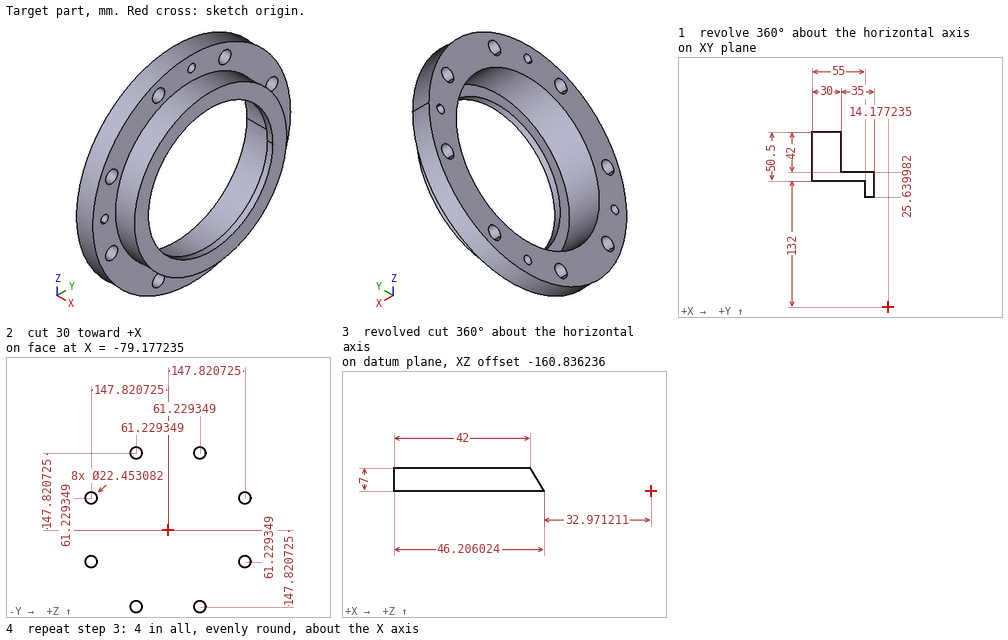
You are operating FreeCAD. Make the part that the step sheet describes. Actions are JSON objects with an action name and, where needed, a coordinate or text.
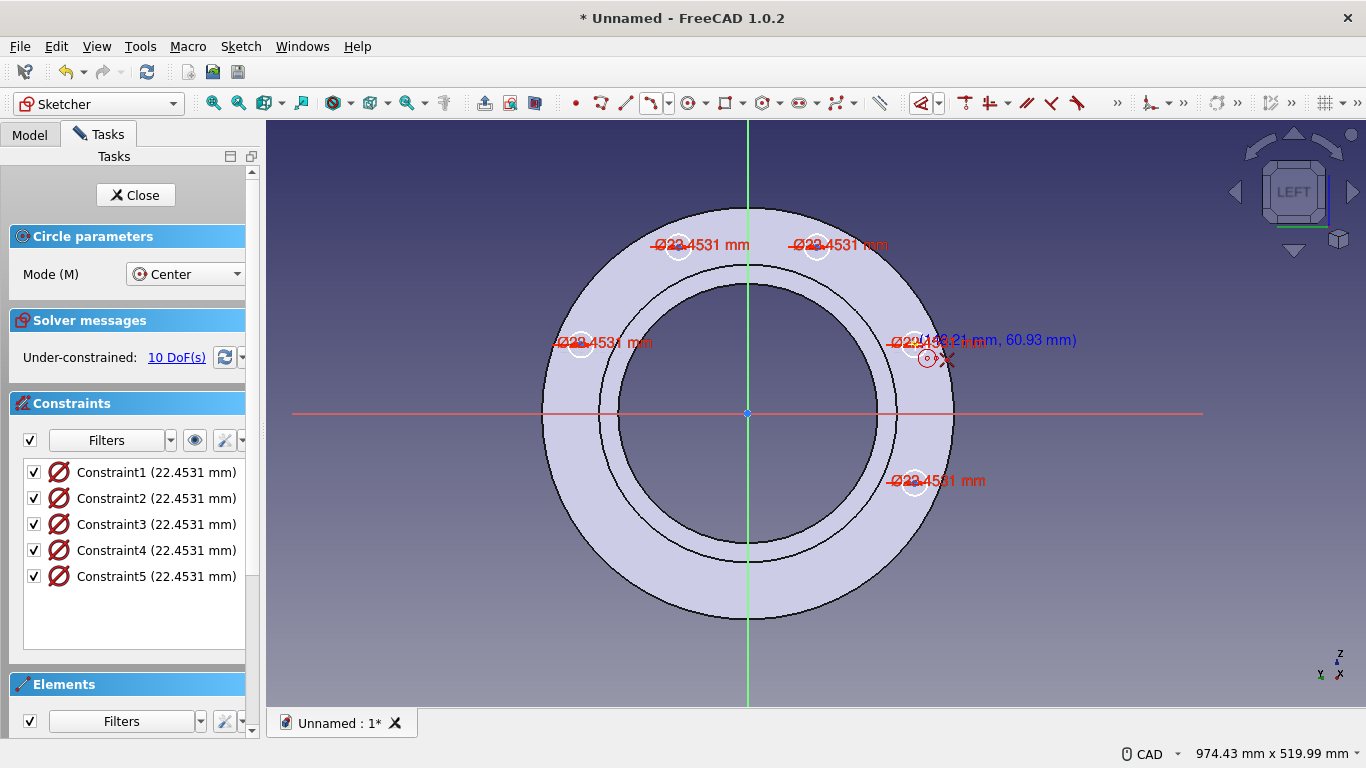
{"action": "scroll", "coordinate": [817, 580], "scroll_direction": "up", "scroll_amount": 3}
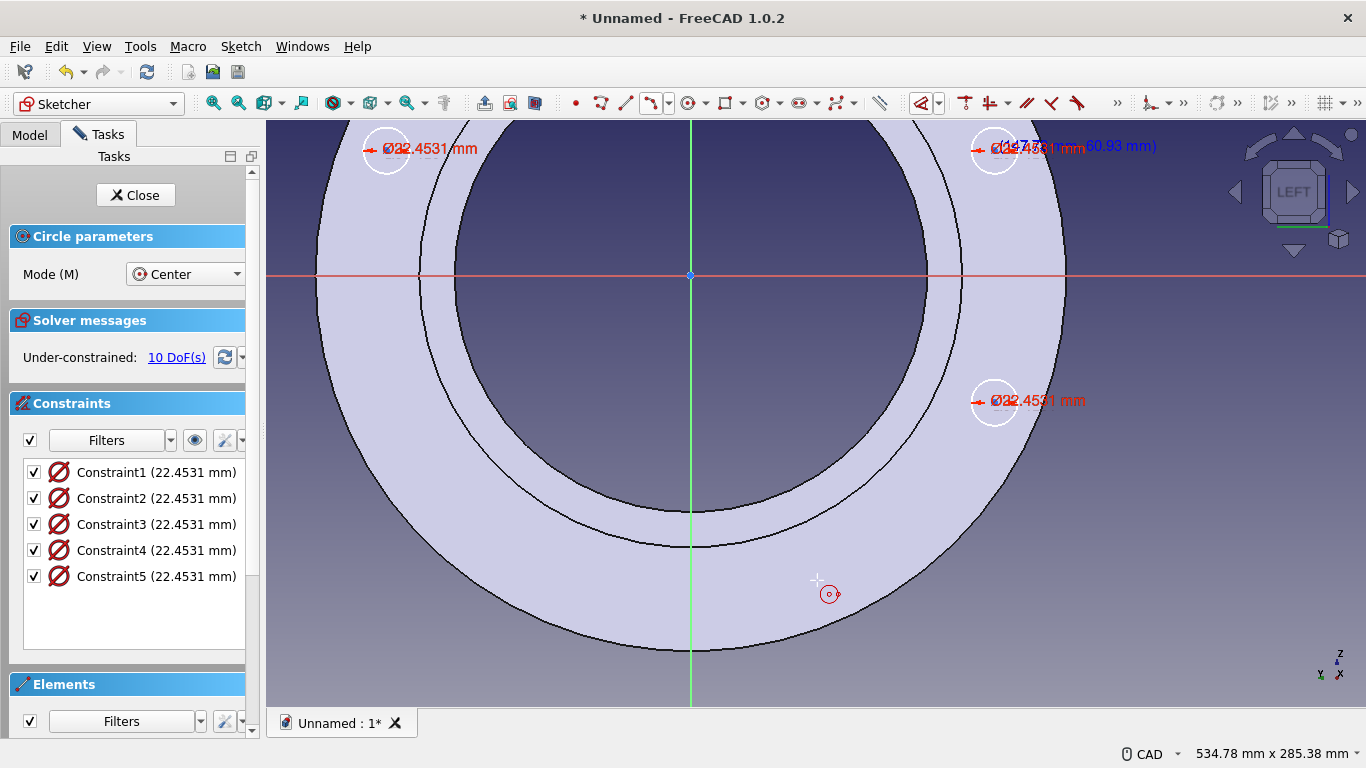
{"action": "left_click", "coordinate": [817, 580]}
{"action": "mouse_move", "coordinate": [833, 564]}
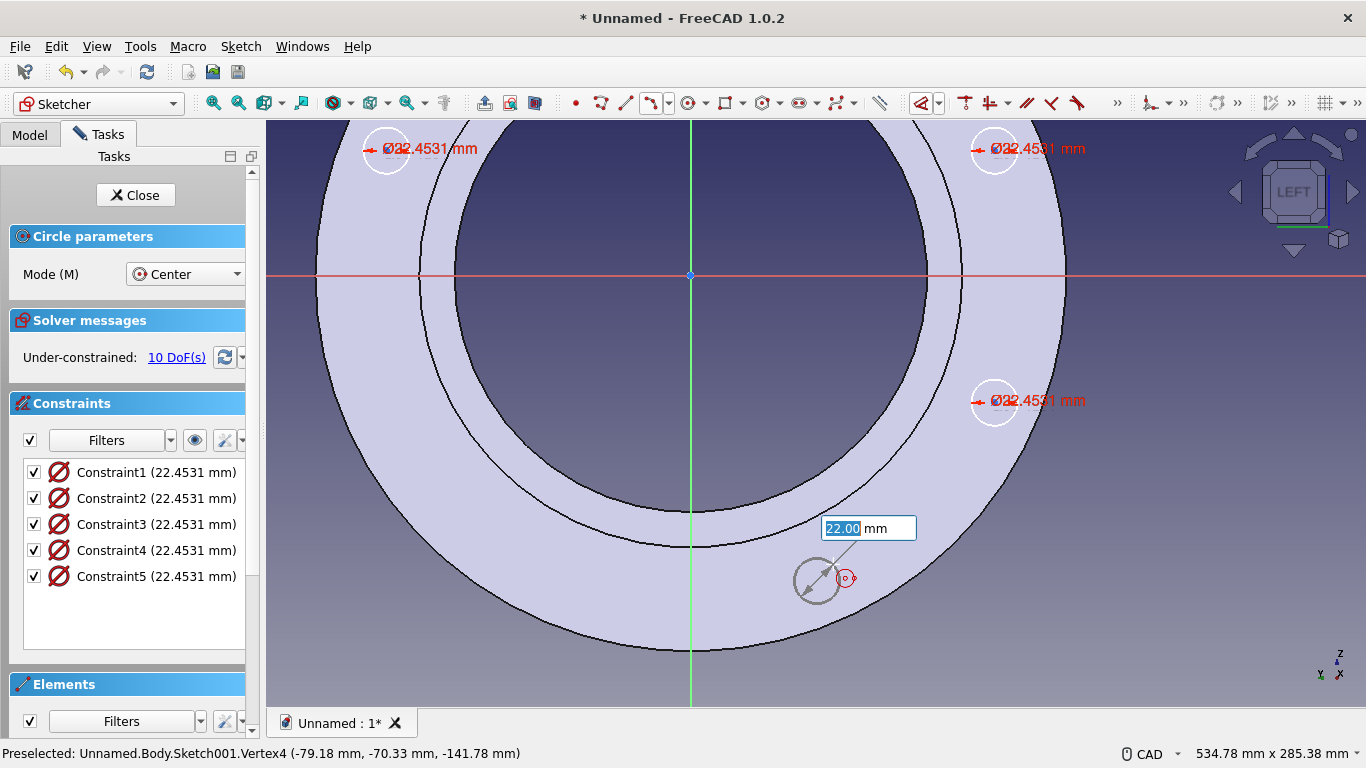
{"action": "type", "text": "22.453082"}
{"action": "key", "text": "Return"}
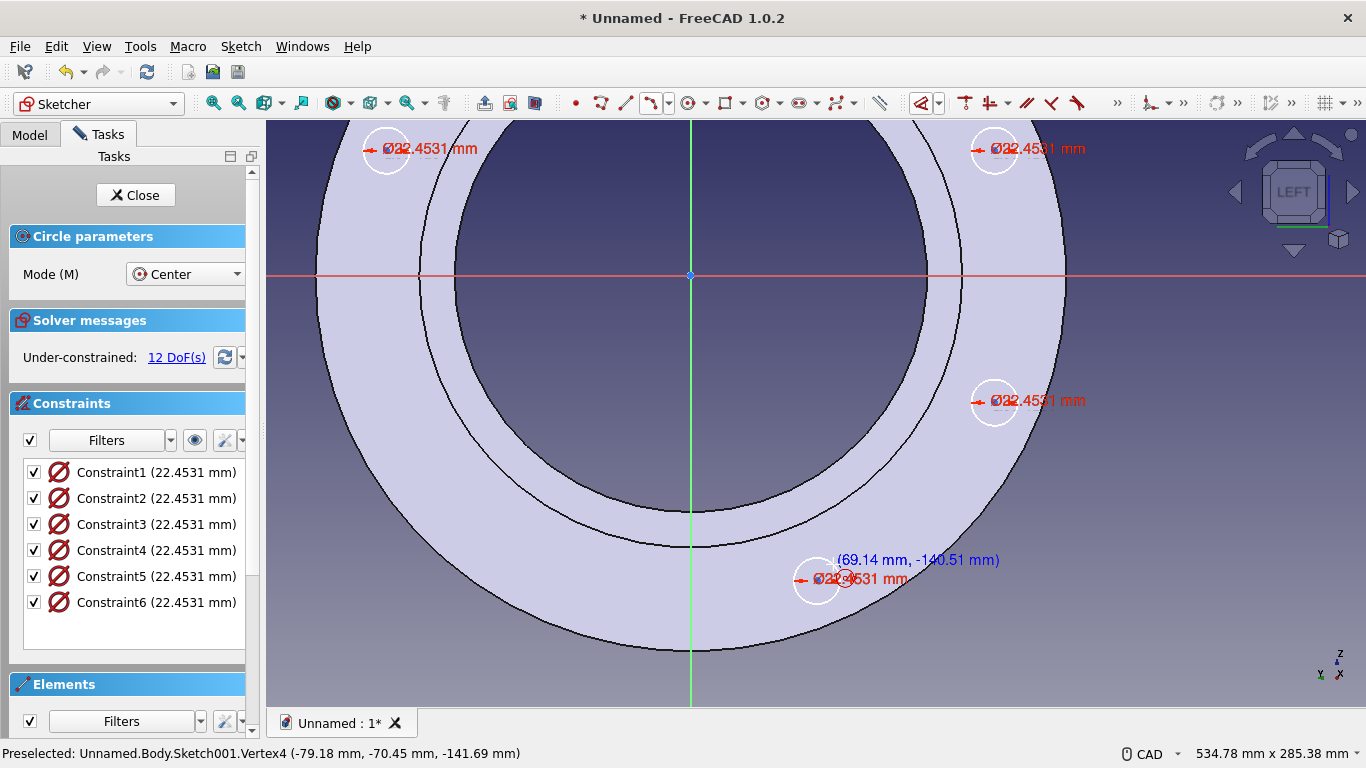
{"action": "left_click", "coordinate": [565, 580]}
{"action": "mouse_move", "coordinate": [581, 564]}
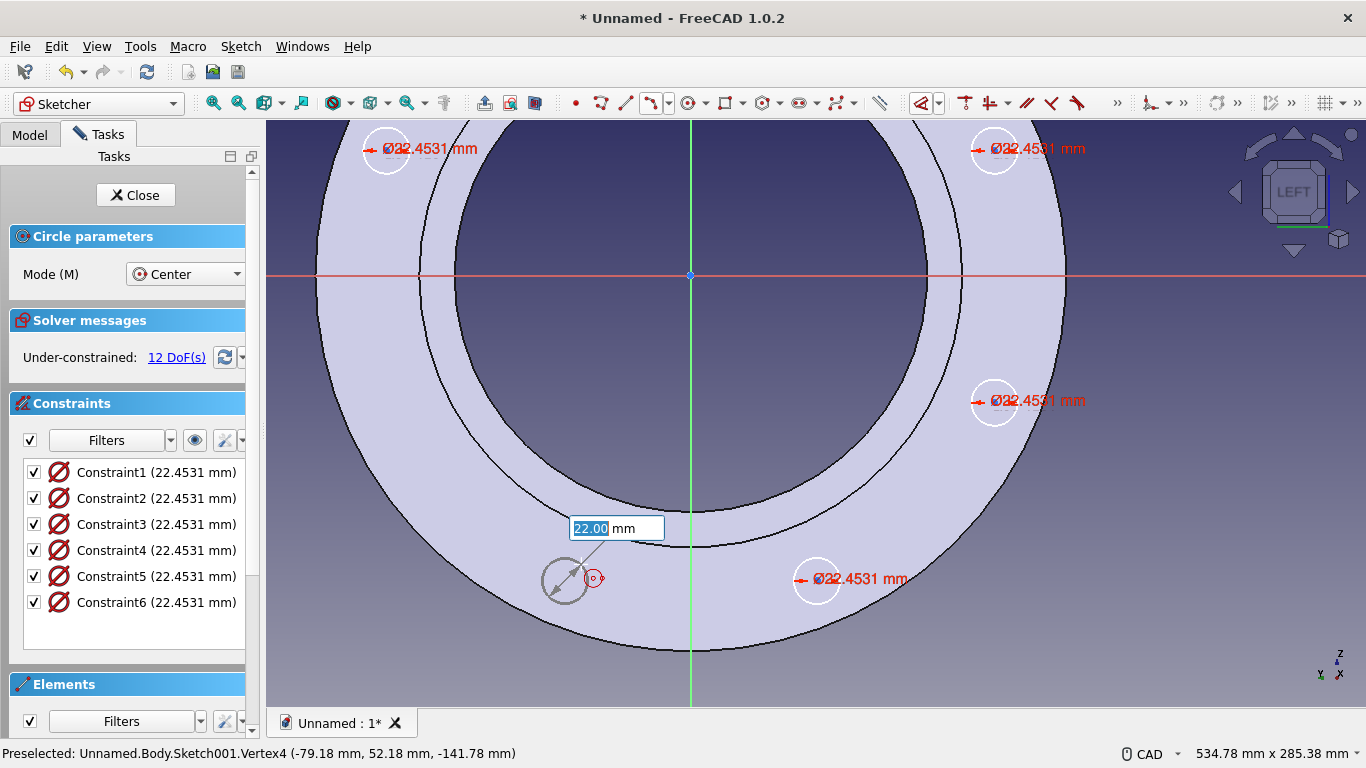
{"action": "type", "text": "22.453082"}
{"action": "key", "text": "Return"}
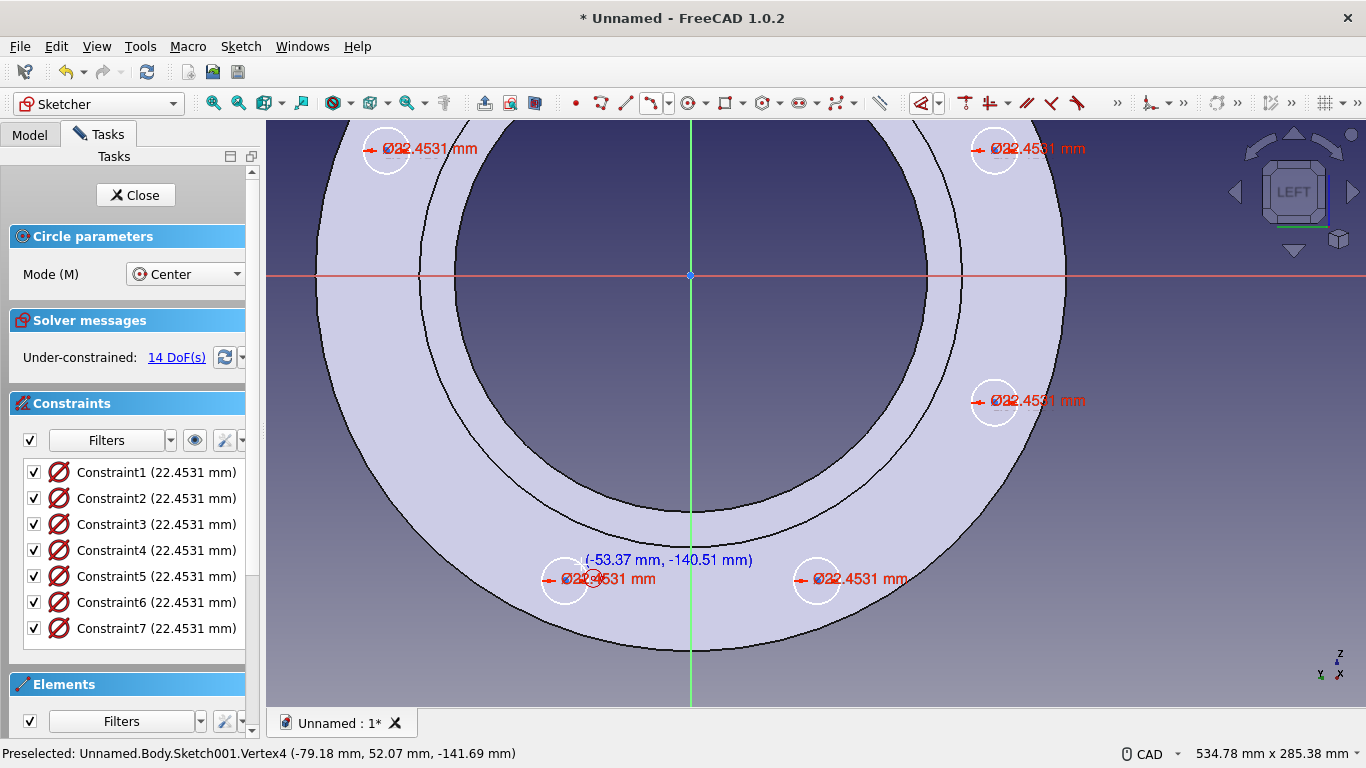
{"action": "left_click", "coordinate": [387, 402]}
{"action": "mouse_move", "coordinate": [403, 386]}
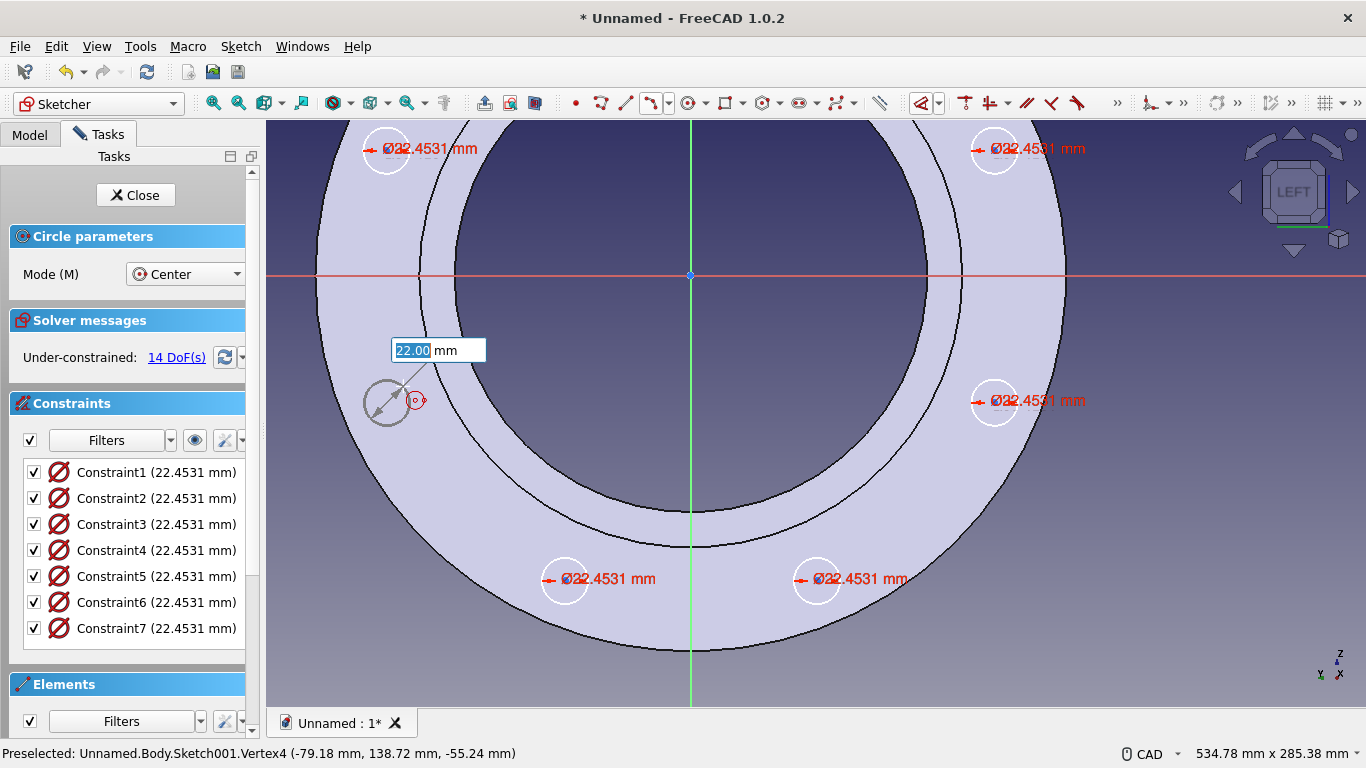
{"action": "type", "text": "22.453082"}
{"action": "key", "text": "Return"}
{"action": "key", "text": "Escape"}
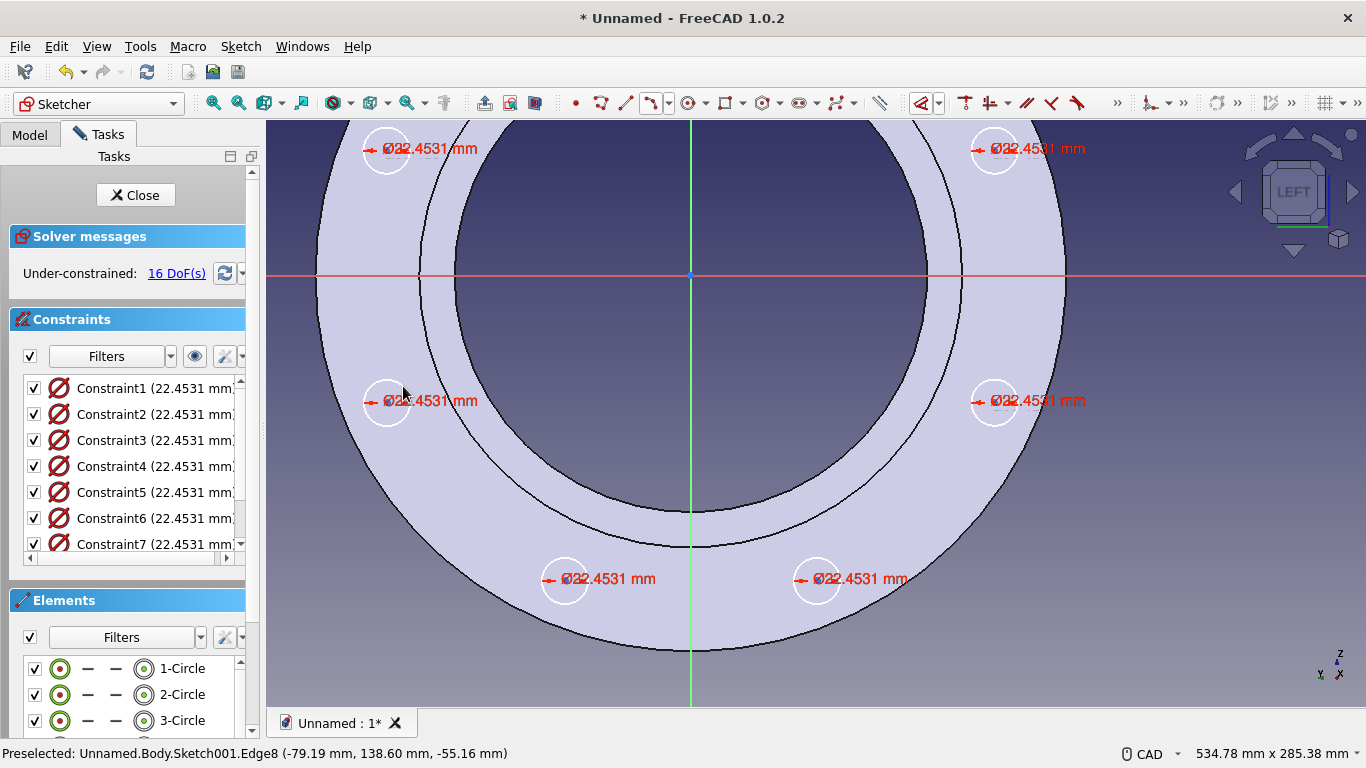
{"action": "scroll", "coordinate": [816, 581], "scroll_direction": "down", "scroll_amount": 3}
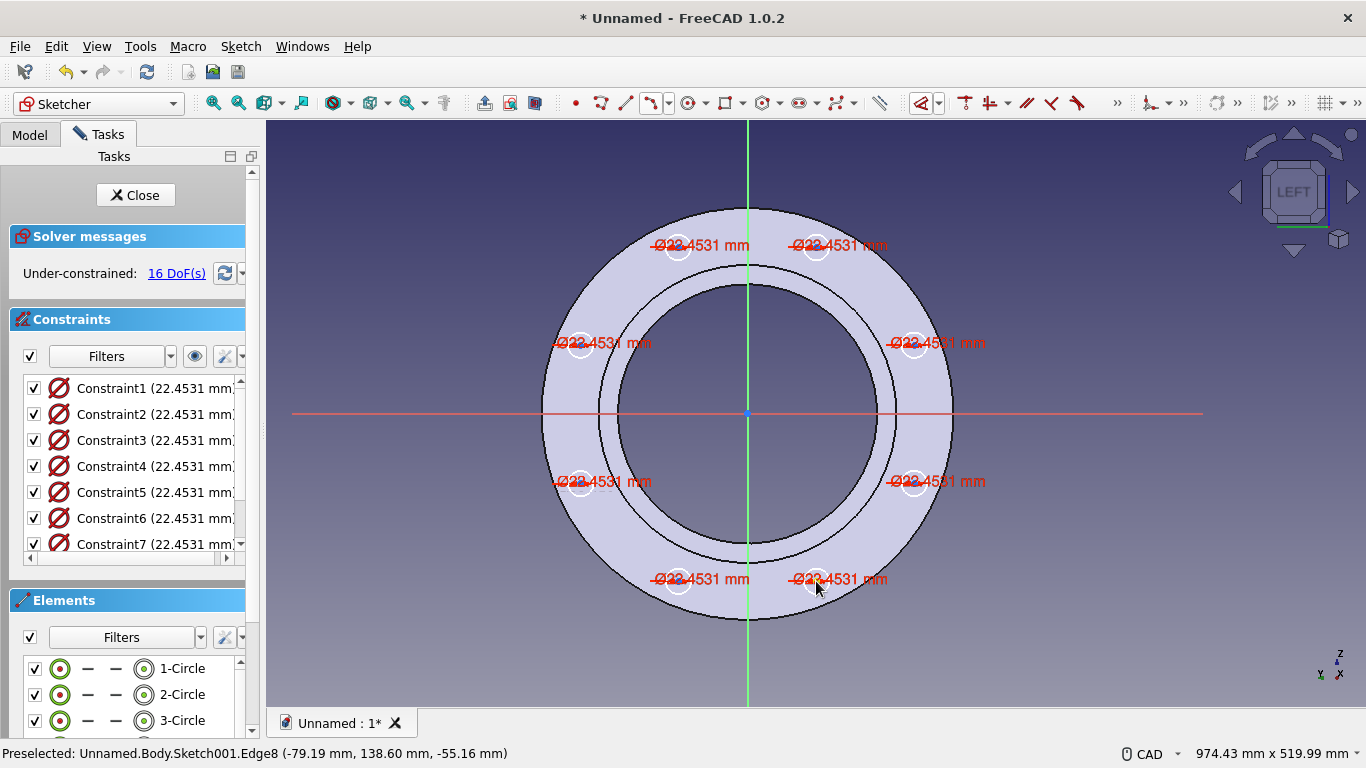
{"action": "left_click", "coordinate": [678, 247]}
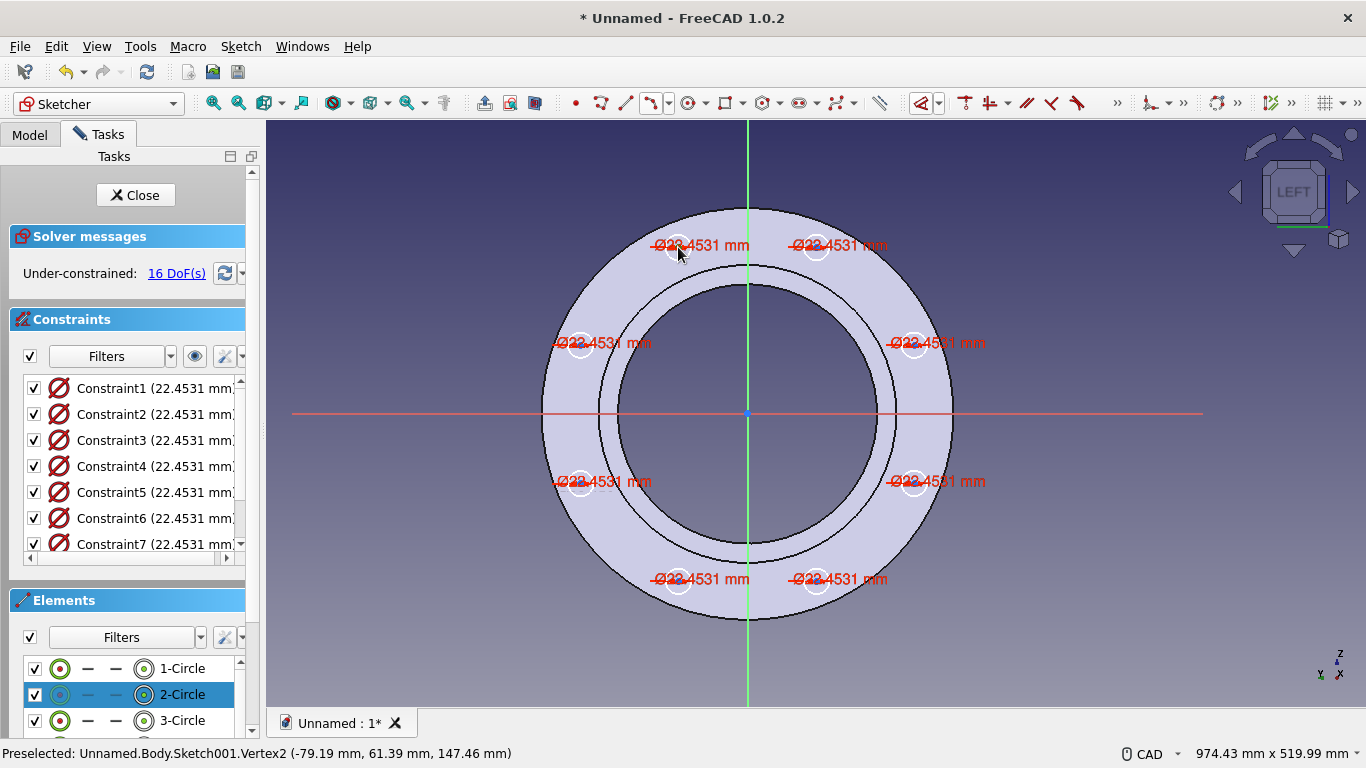
{"action": "left_click", "coordinate": [817, 247]}